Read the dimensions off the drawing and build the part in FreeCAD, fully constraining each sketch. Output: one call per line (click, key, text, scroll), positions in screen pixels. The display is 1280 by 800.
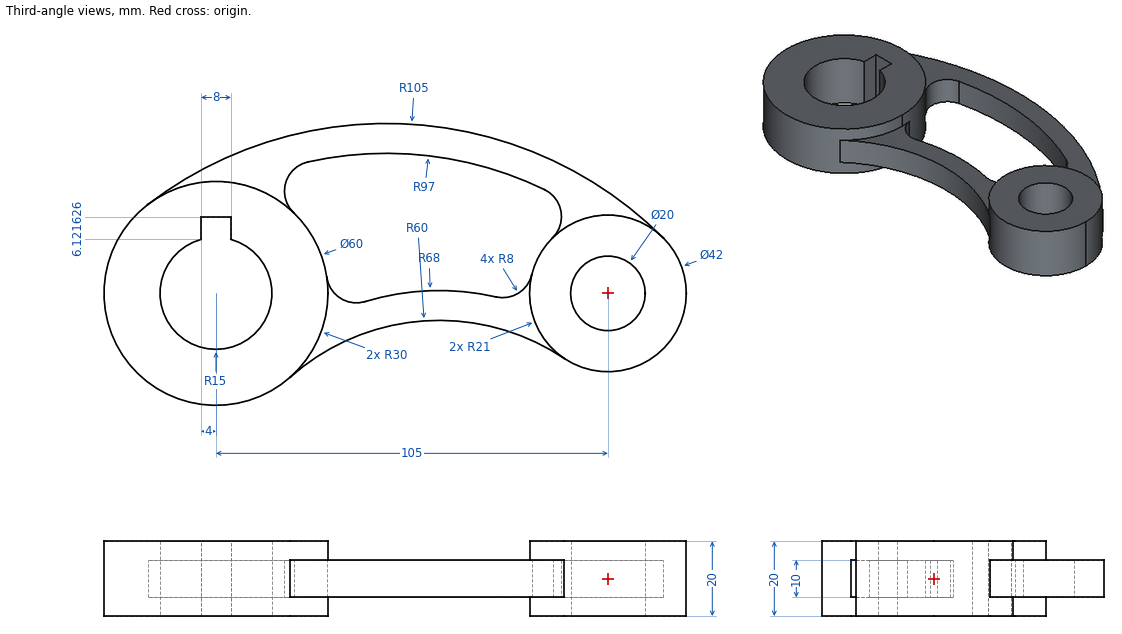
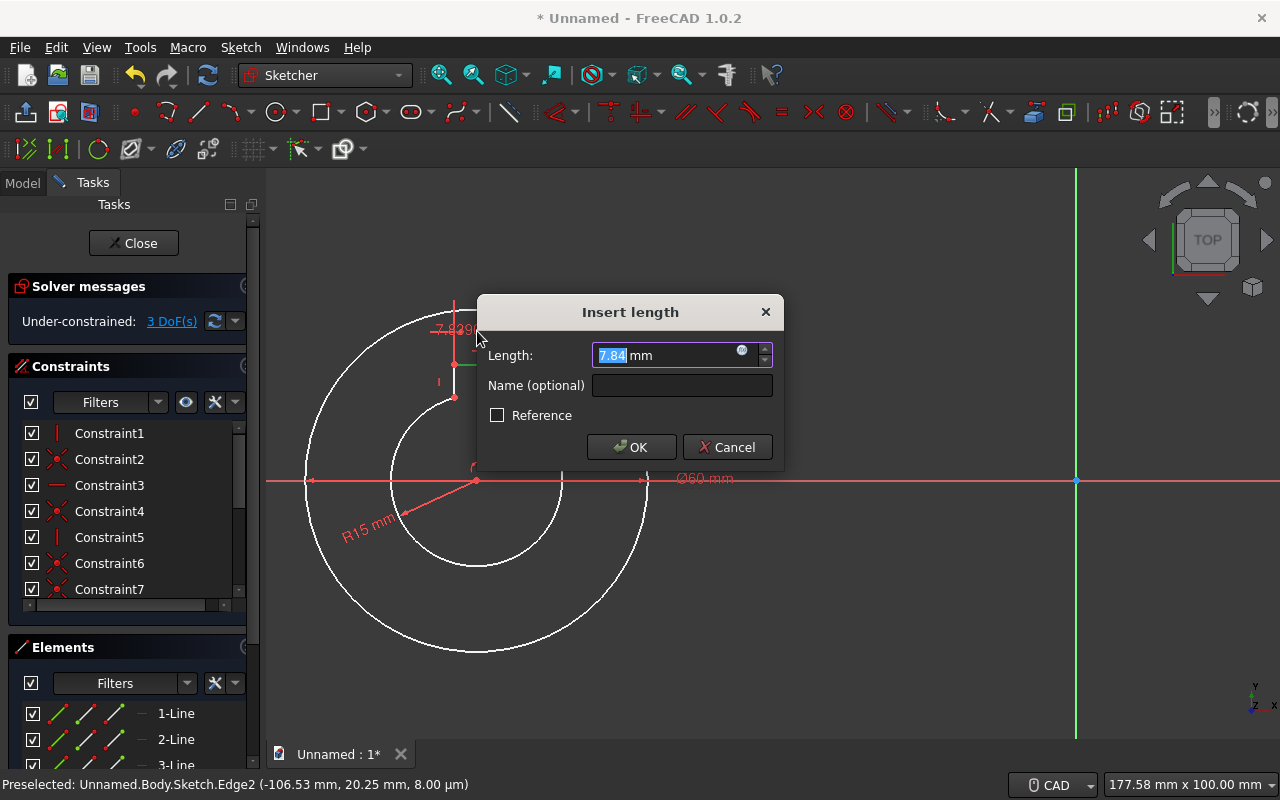
text(8)
key(Return)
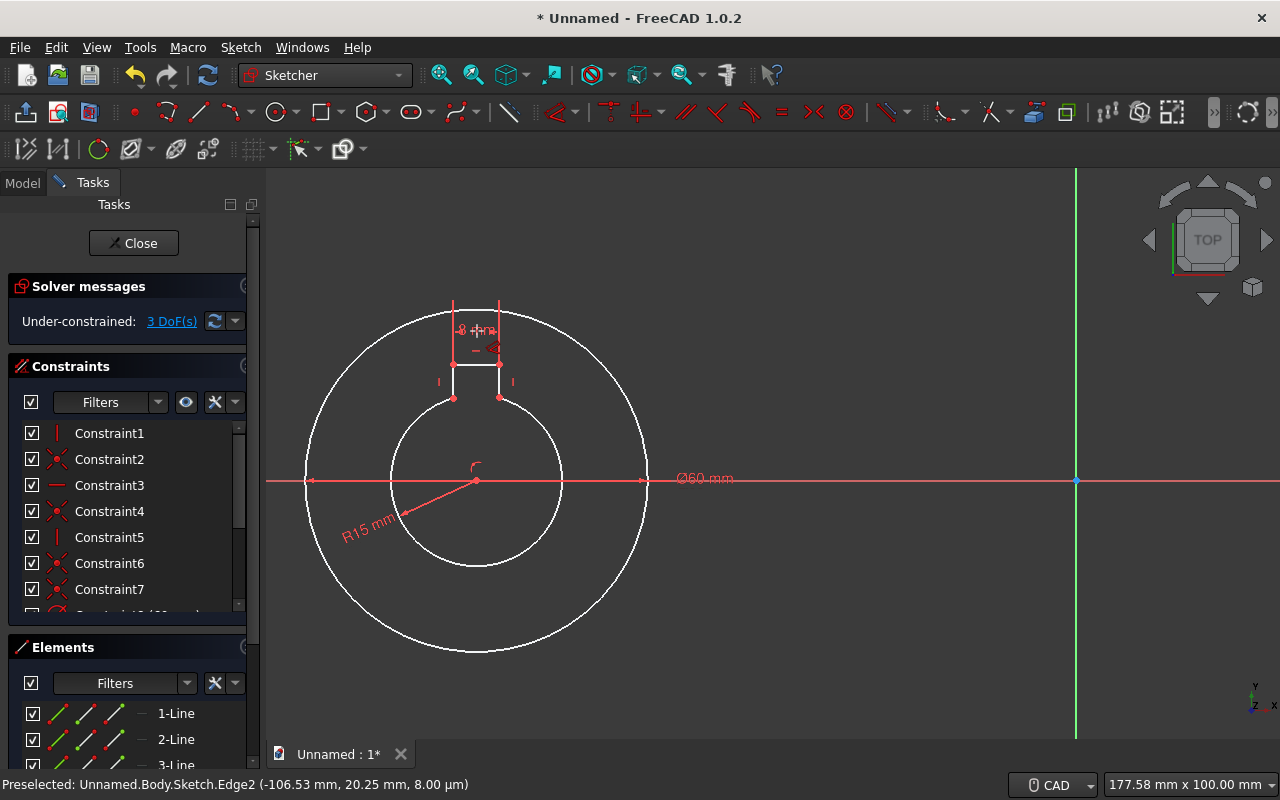
scroll(453, 398, up, 3)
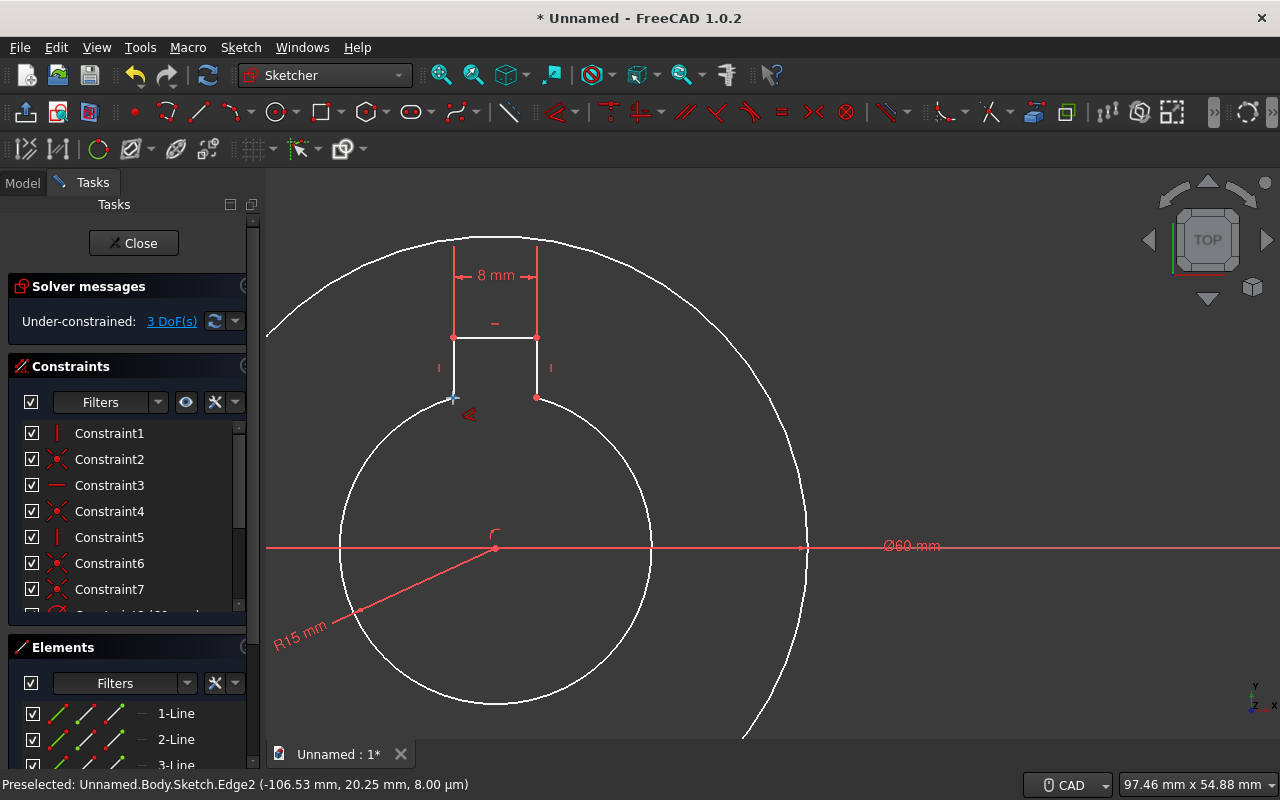
click(454, 398)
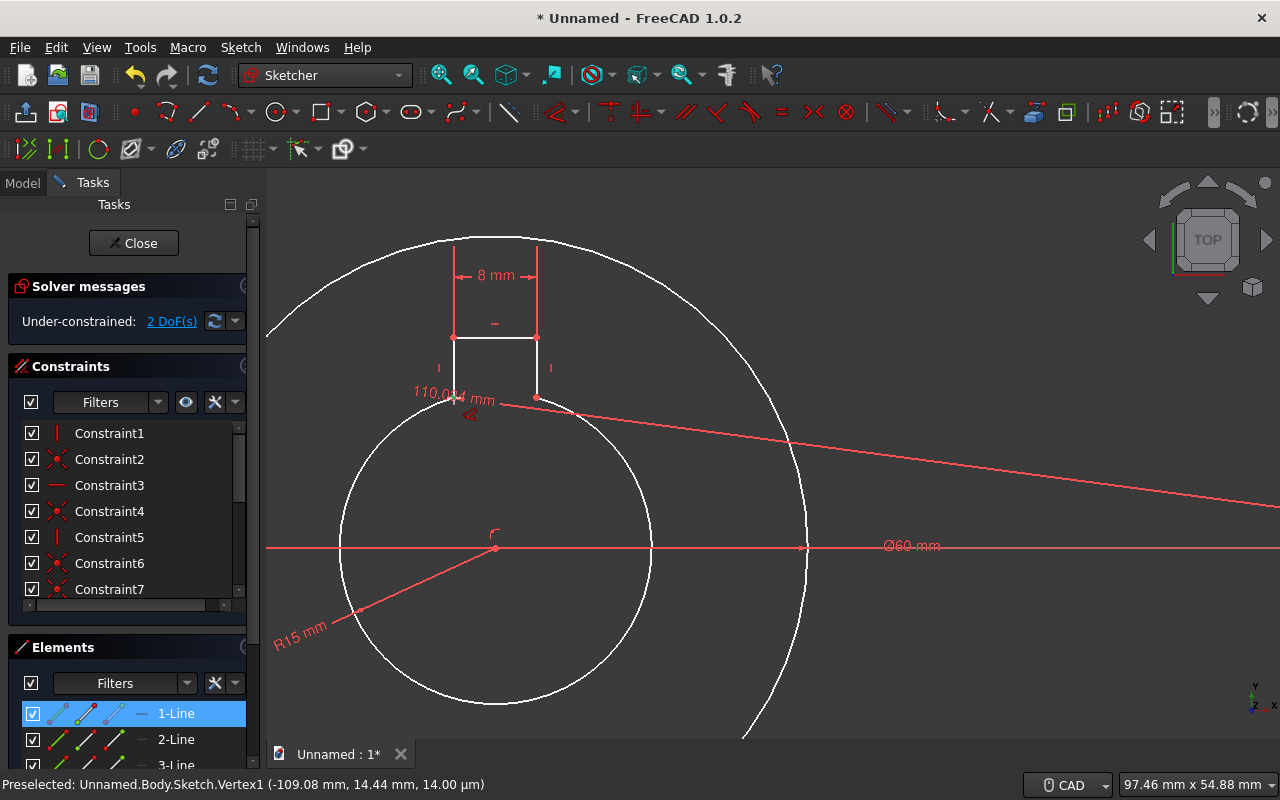
click(496, 548)
click(475, 364)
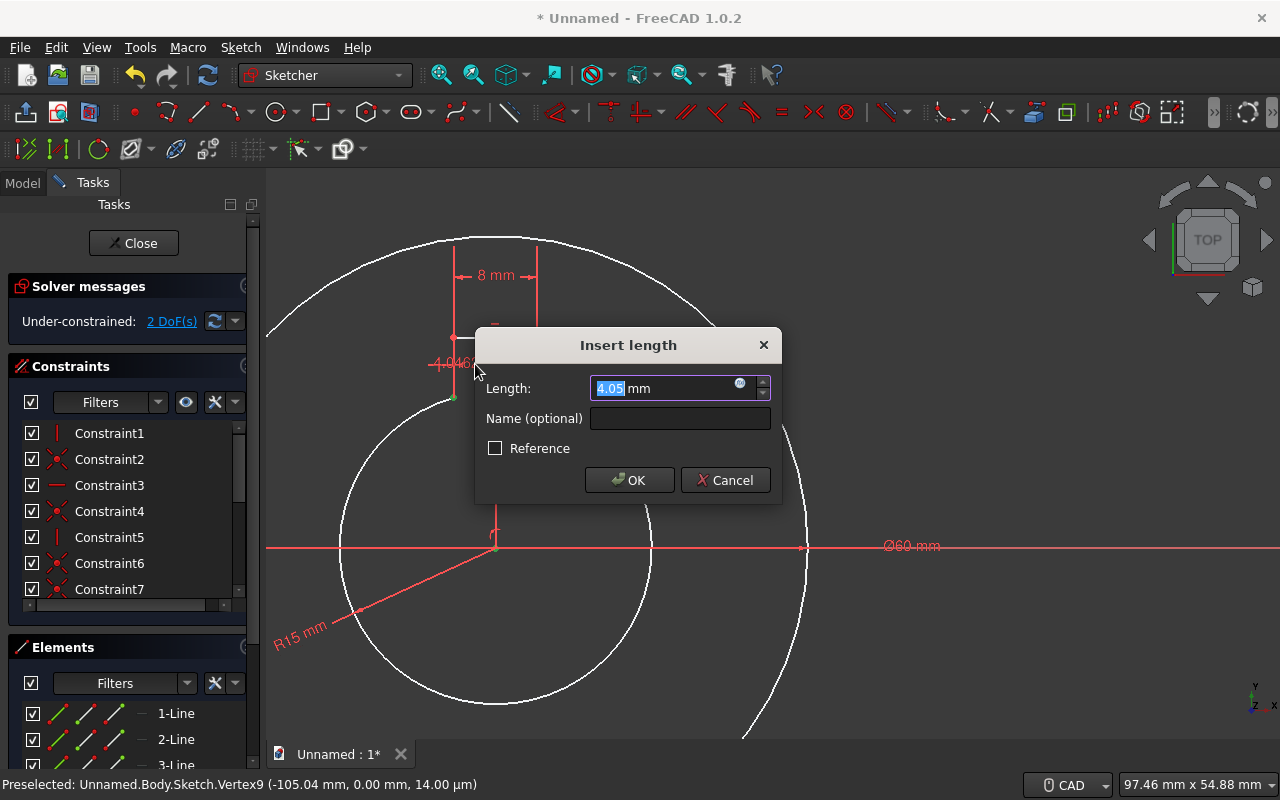
text(4)
key(Return)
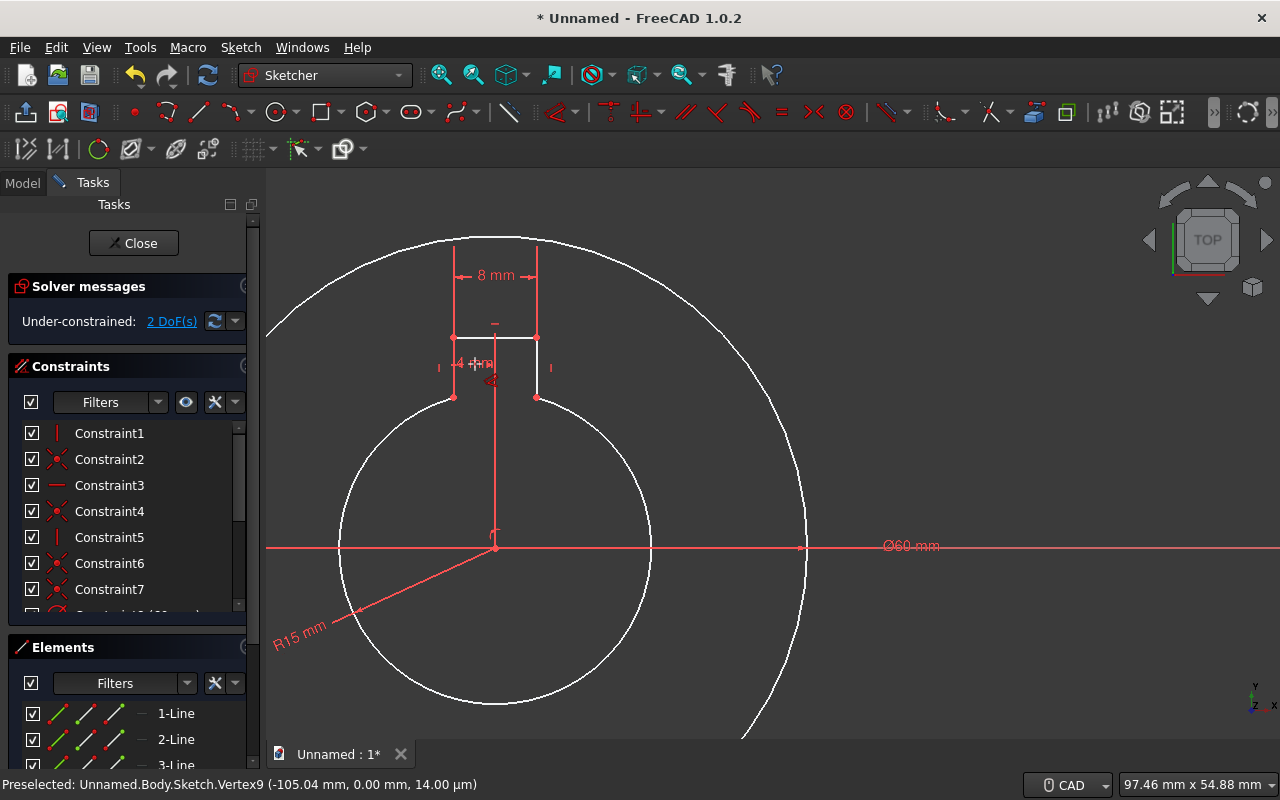
click(495, 548)
click(663, 582)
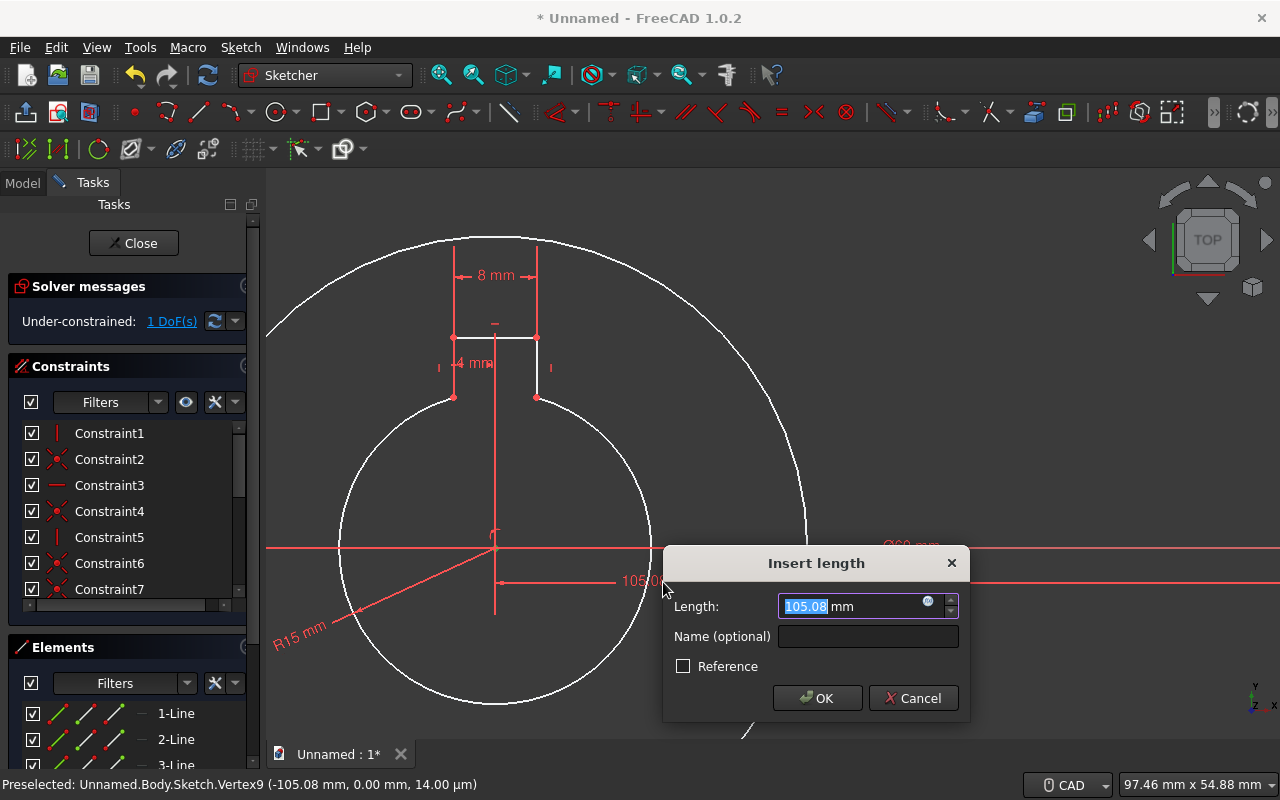
text(105)
key(Return)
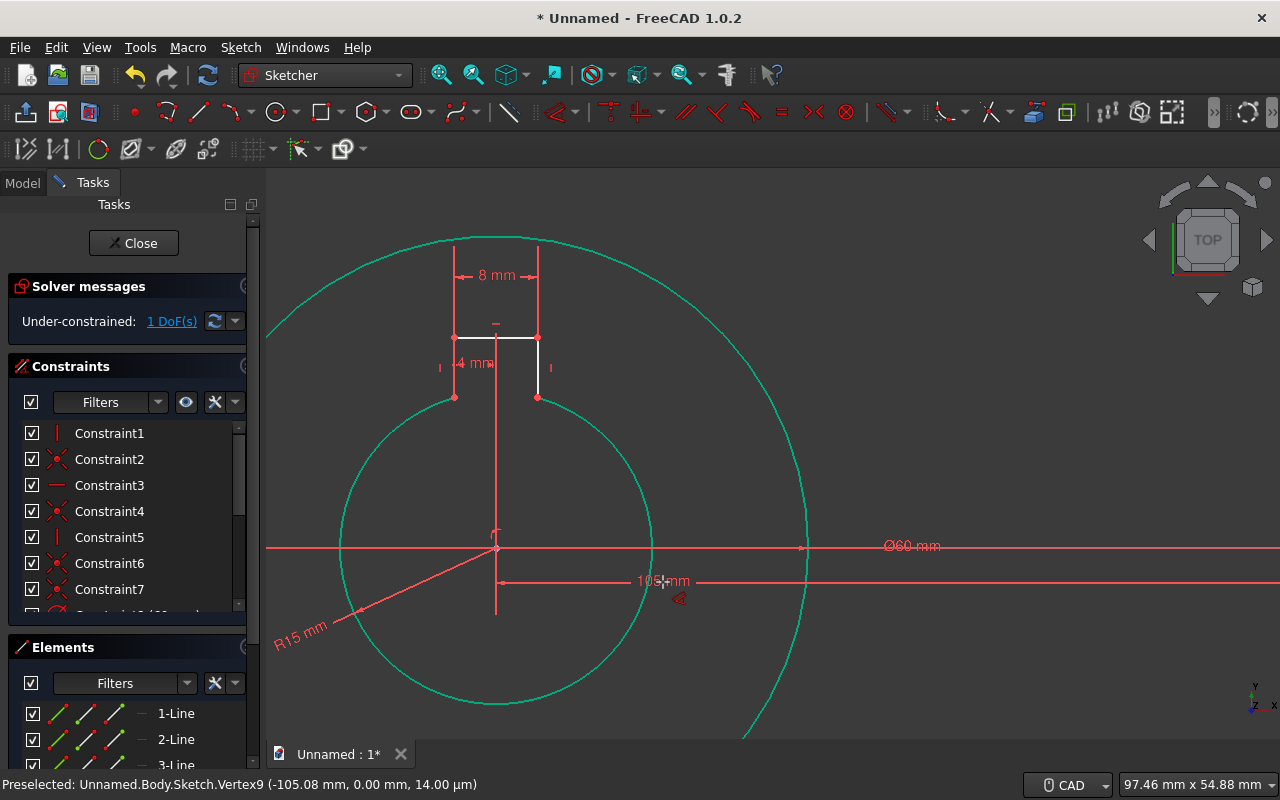
click(454, 380)
click(420, 389)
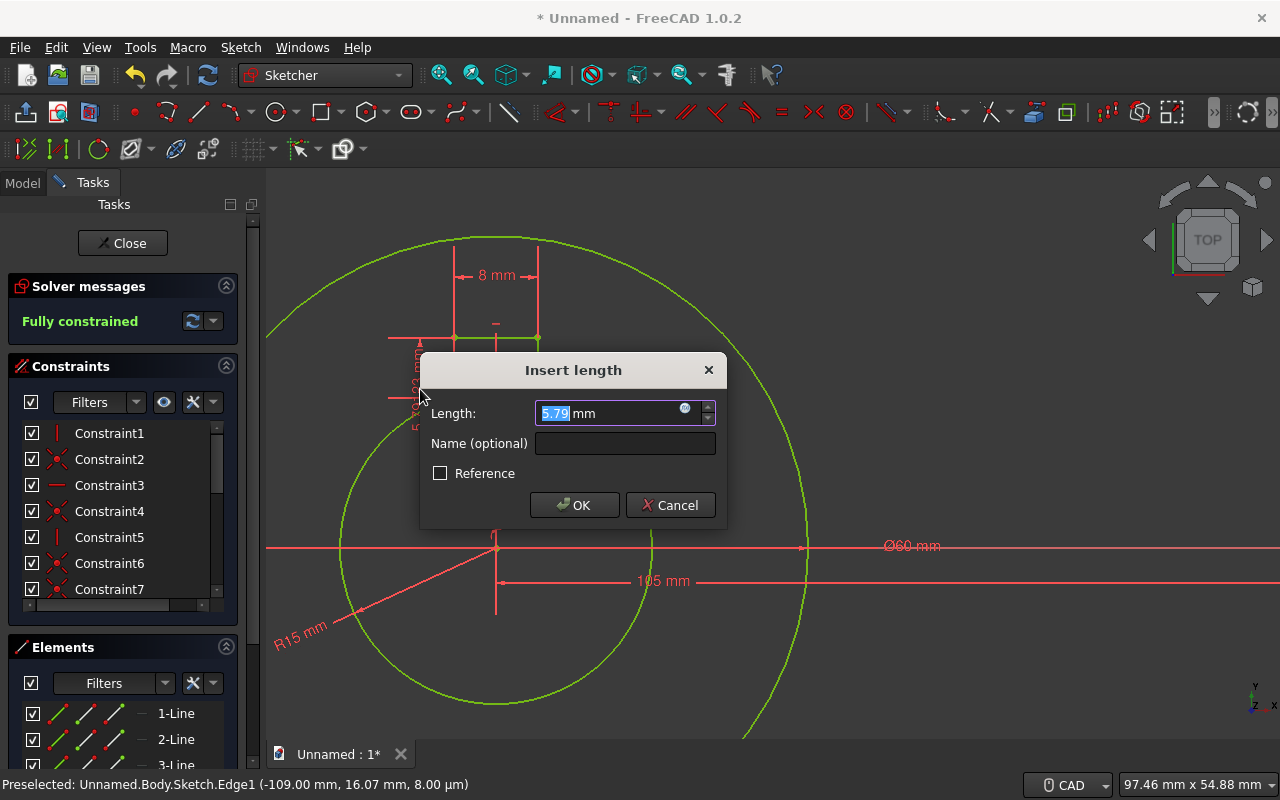
text(6.121626)
key(Return)
key(Escape)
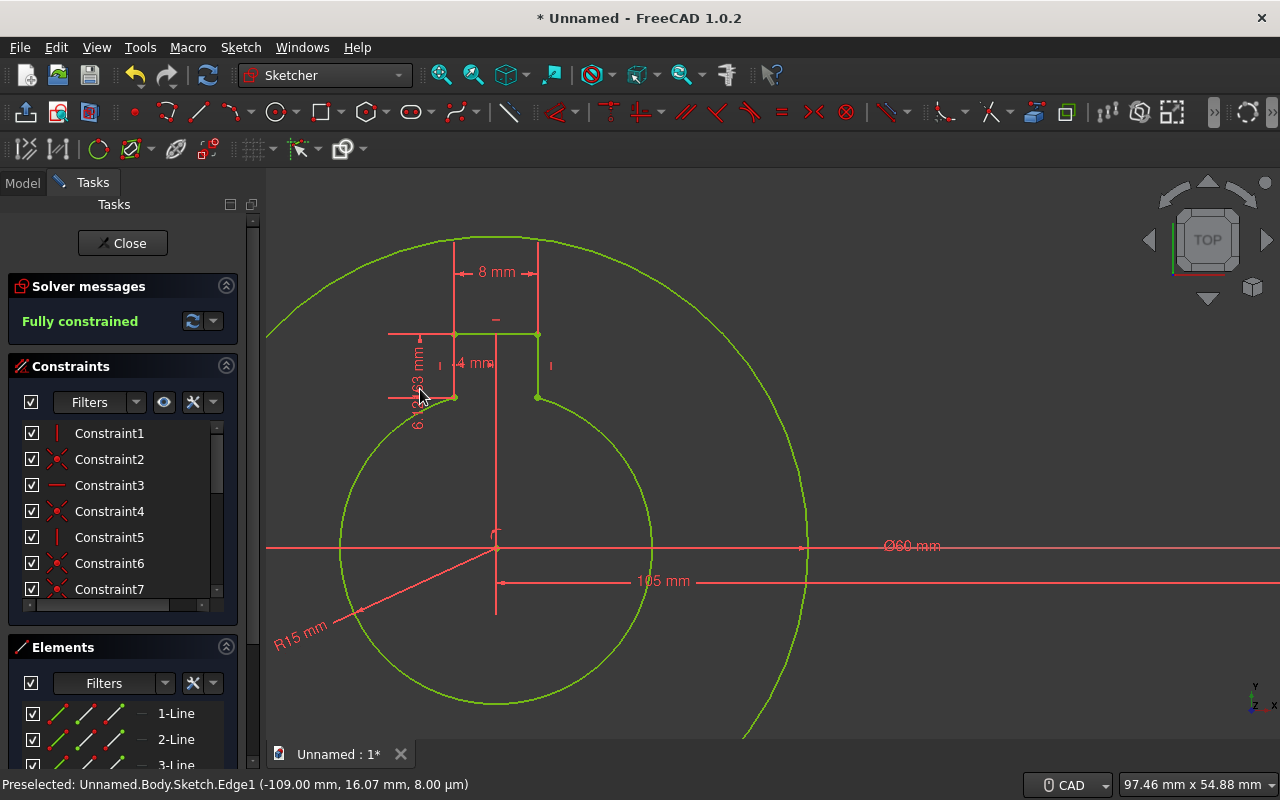
click(123, 243)